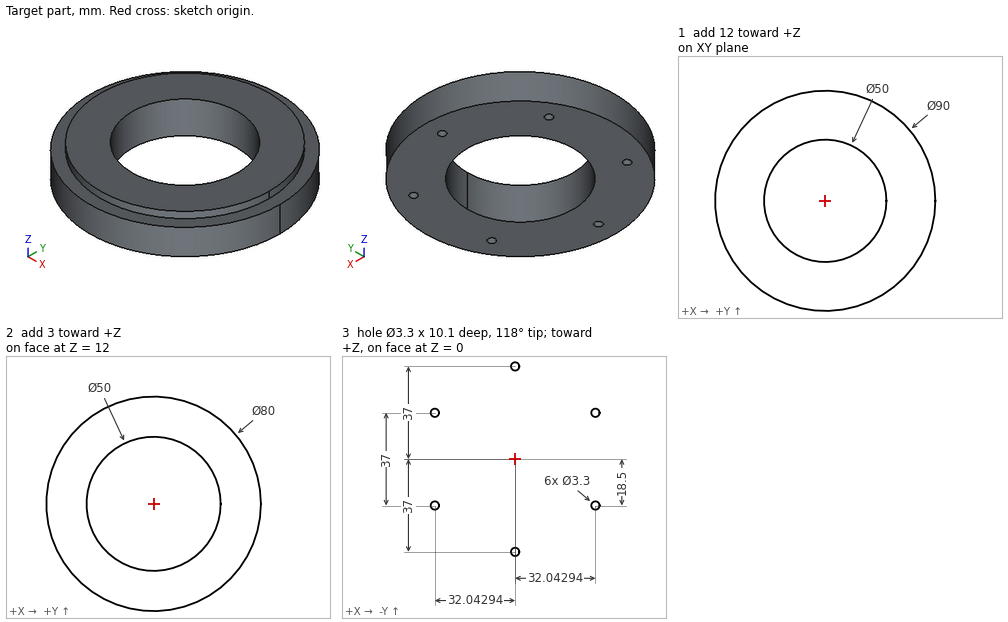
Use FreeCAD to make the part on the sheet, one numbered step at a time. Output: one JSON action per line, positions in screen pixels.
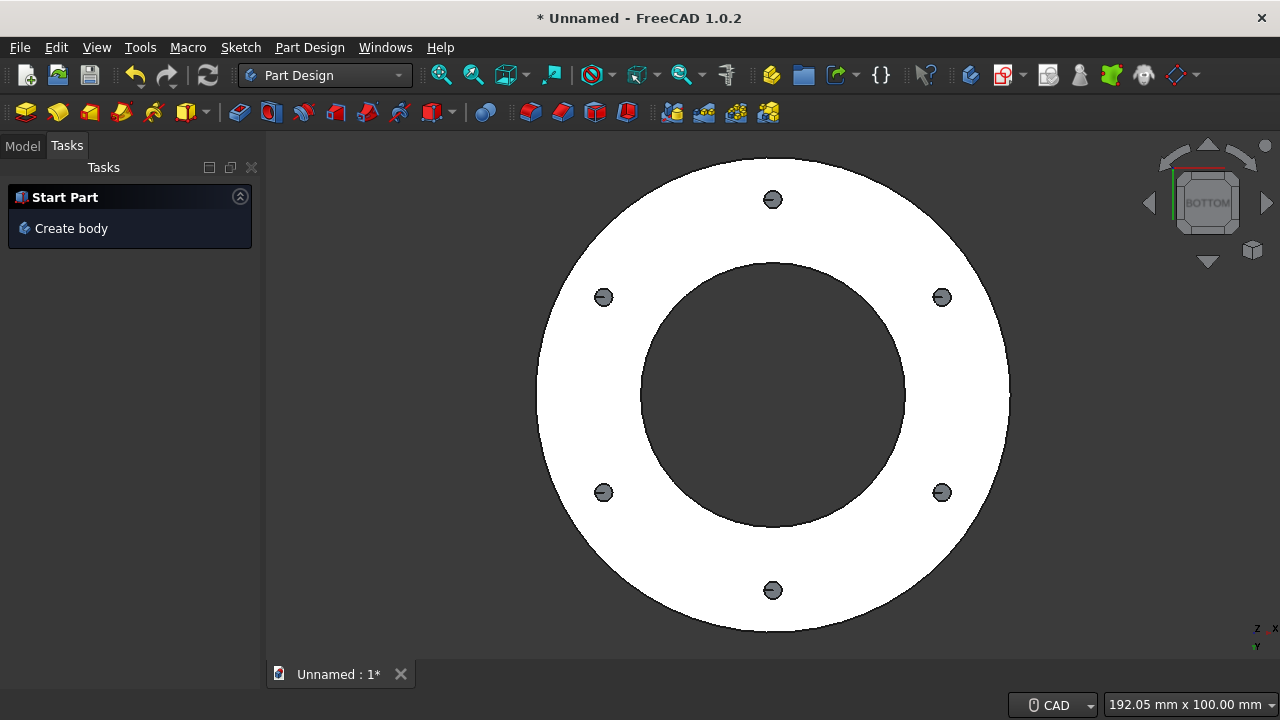
{"action": "key", "text": "0"}